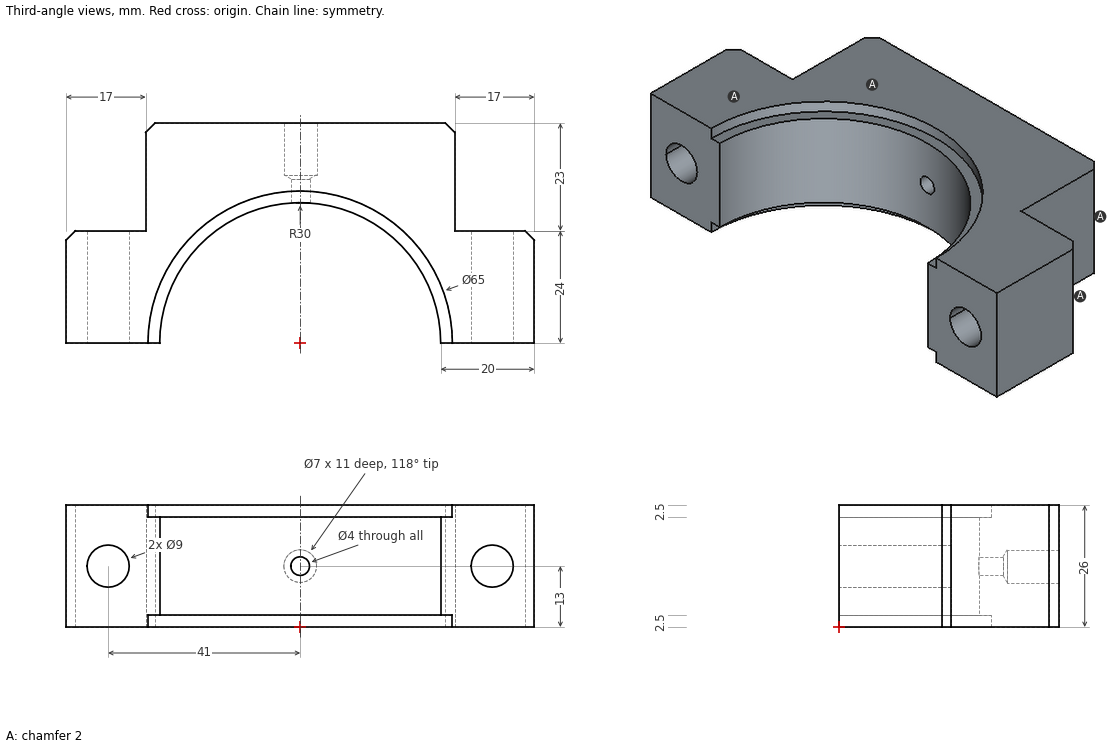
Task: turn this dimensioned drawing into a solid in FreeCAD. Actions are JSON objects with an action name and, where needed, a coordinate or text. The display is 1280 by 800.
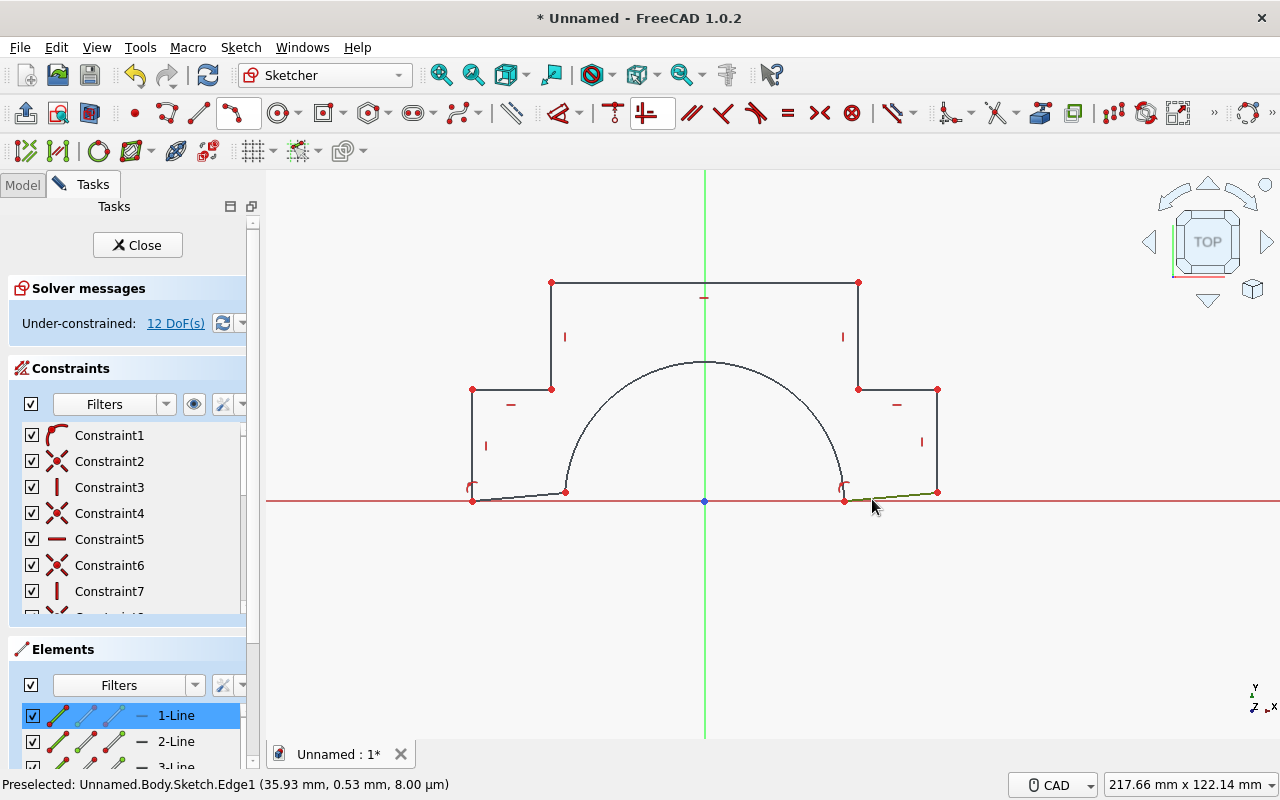
{"action": "key", "text": "h"}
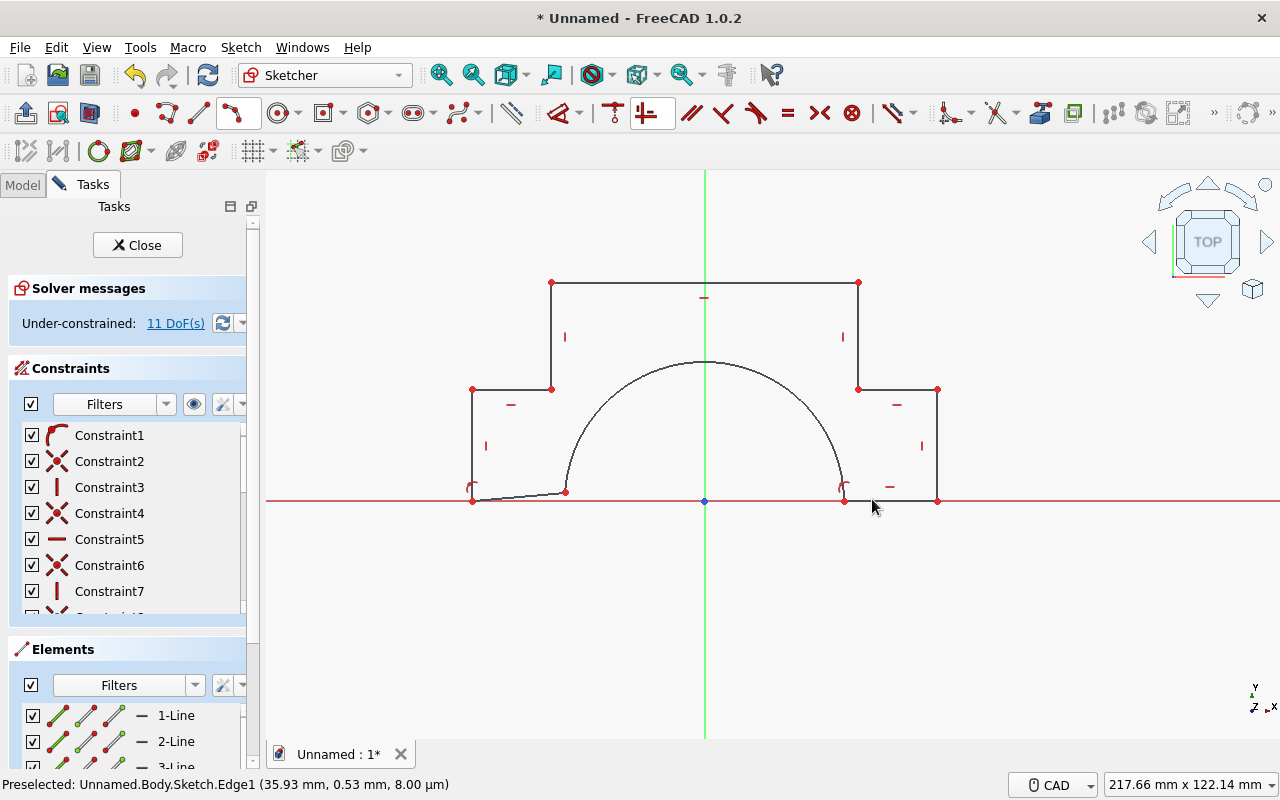
{"action": "left_click", "coordinate": [500, 499]}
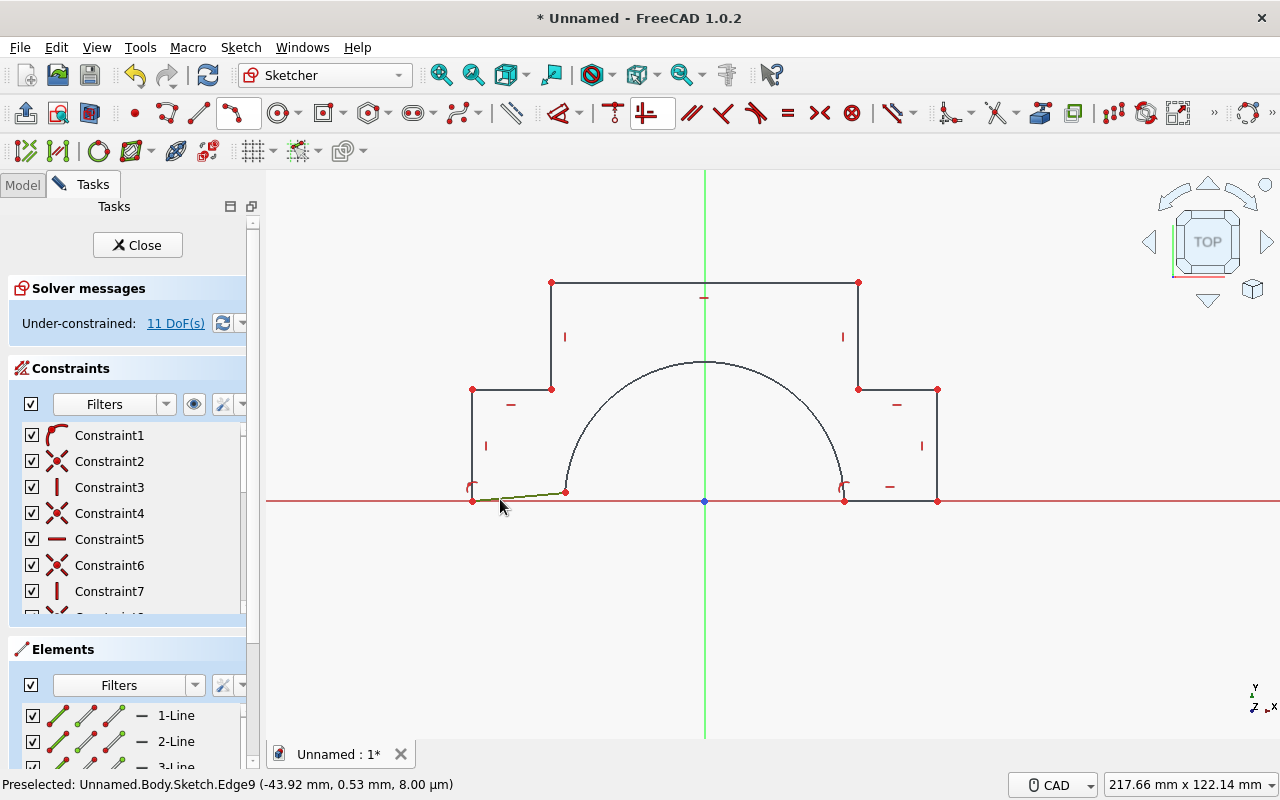
{"action": "key", "text": "h"}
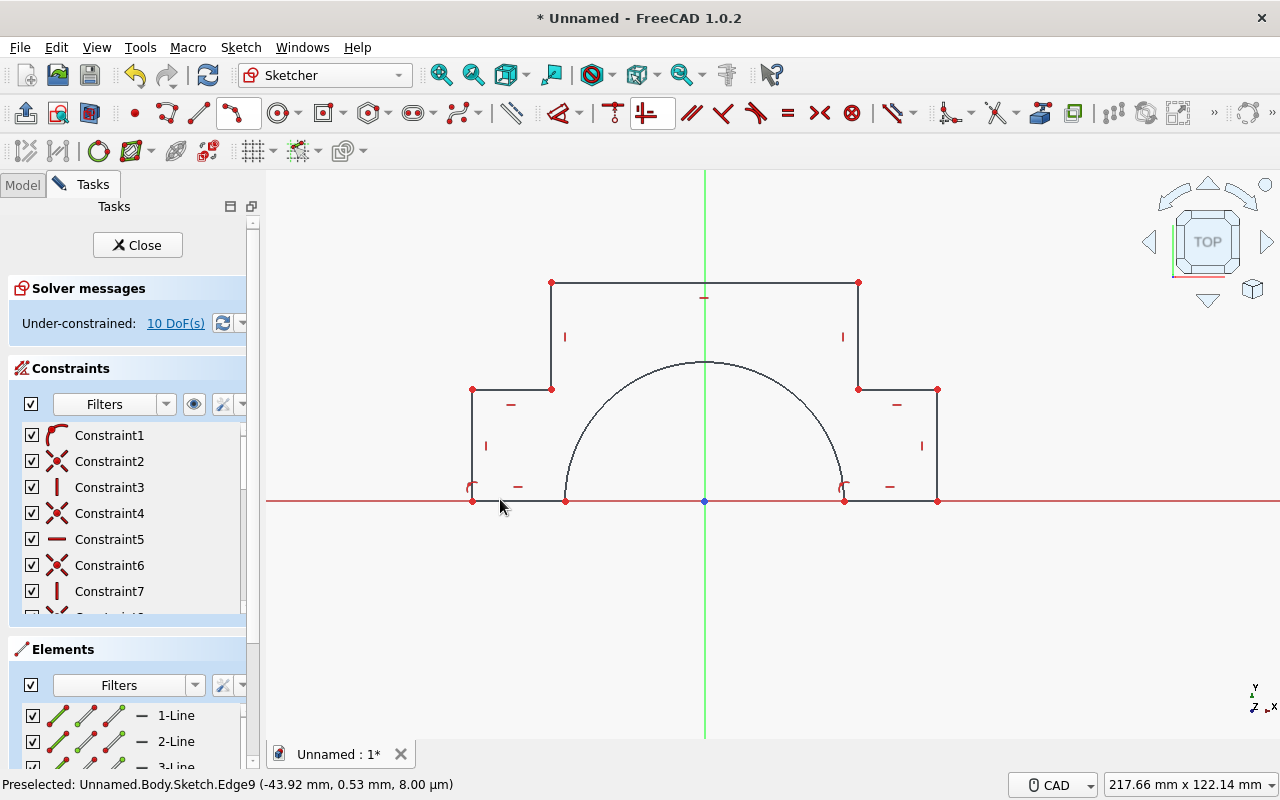
{"action": "left_click_drag", "start_coordinate": [695, 491], "coordinate": [715, 512]}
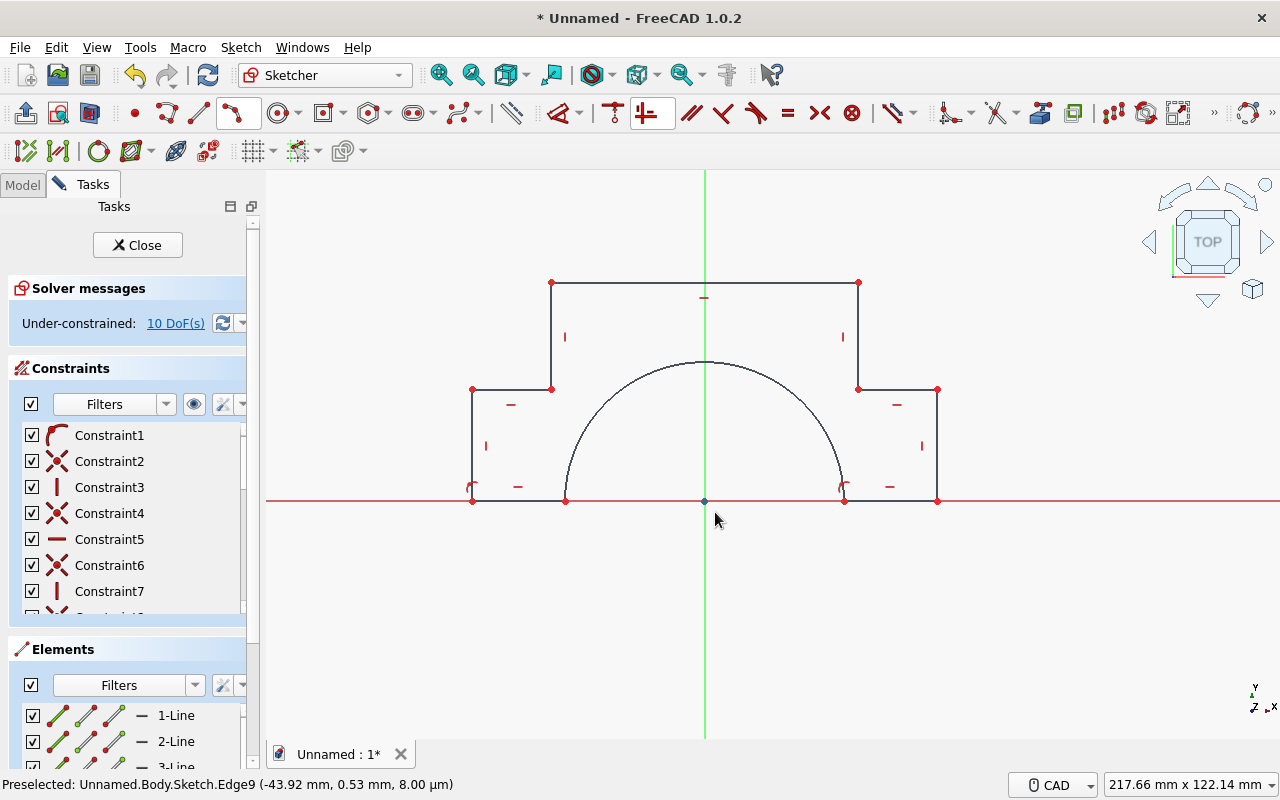
{"action": "key", "text": "c"}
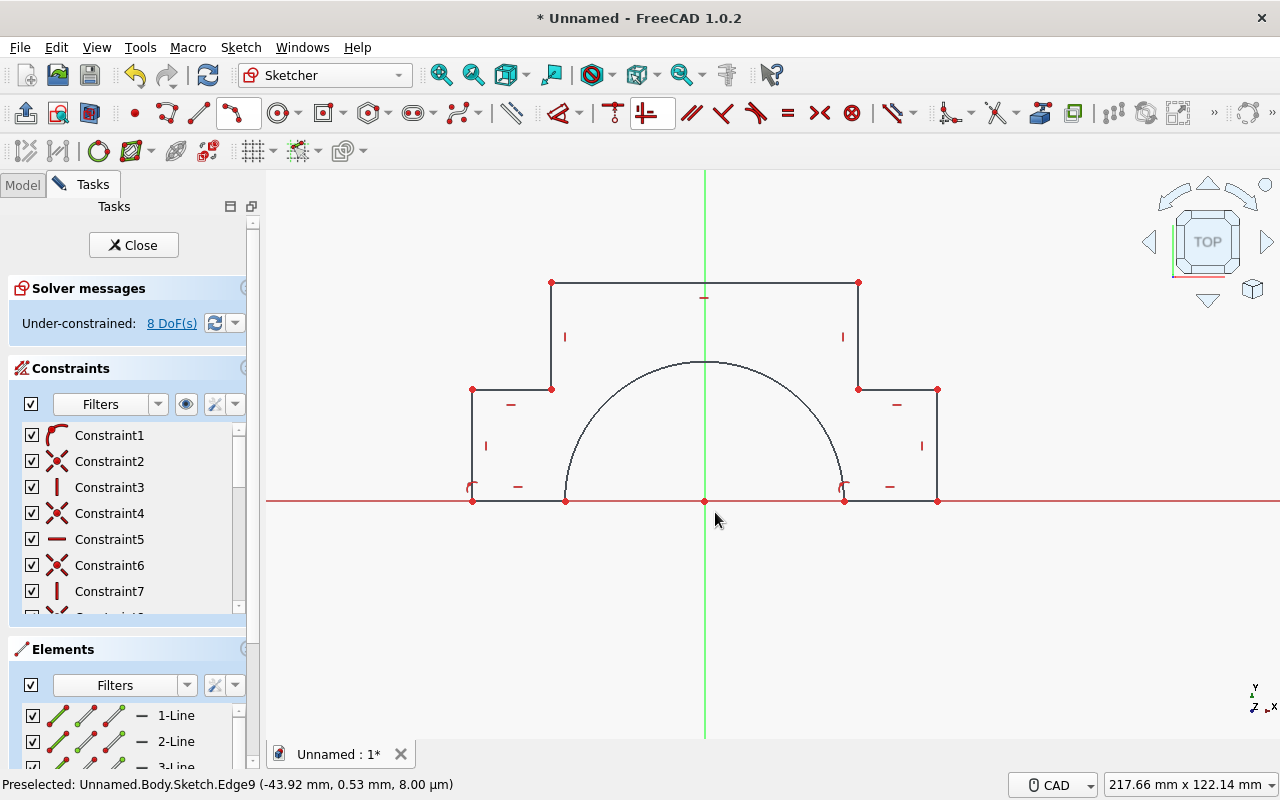
{"action": "left_click", "coordinate": [858, 390]}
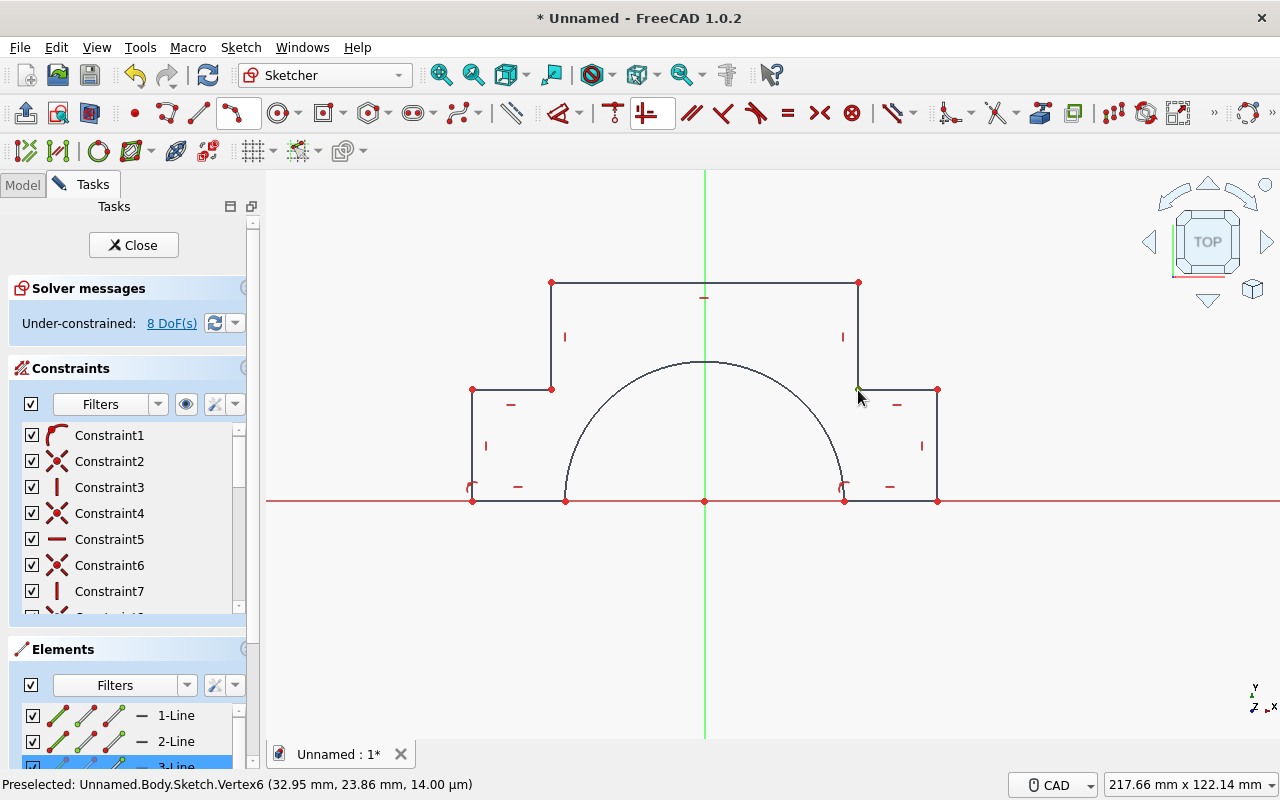
{"action": "left_click", "coordinate": [551, 390]}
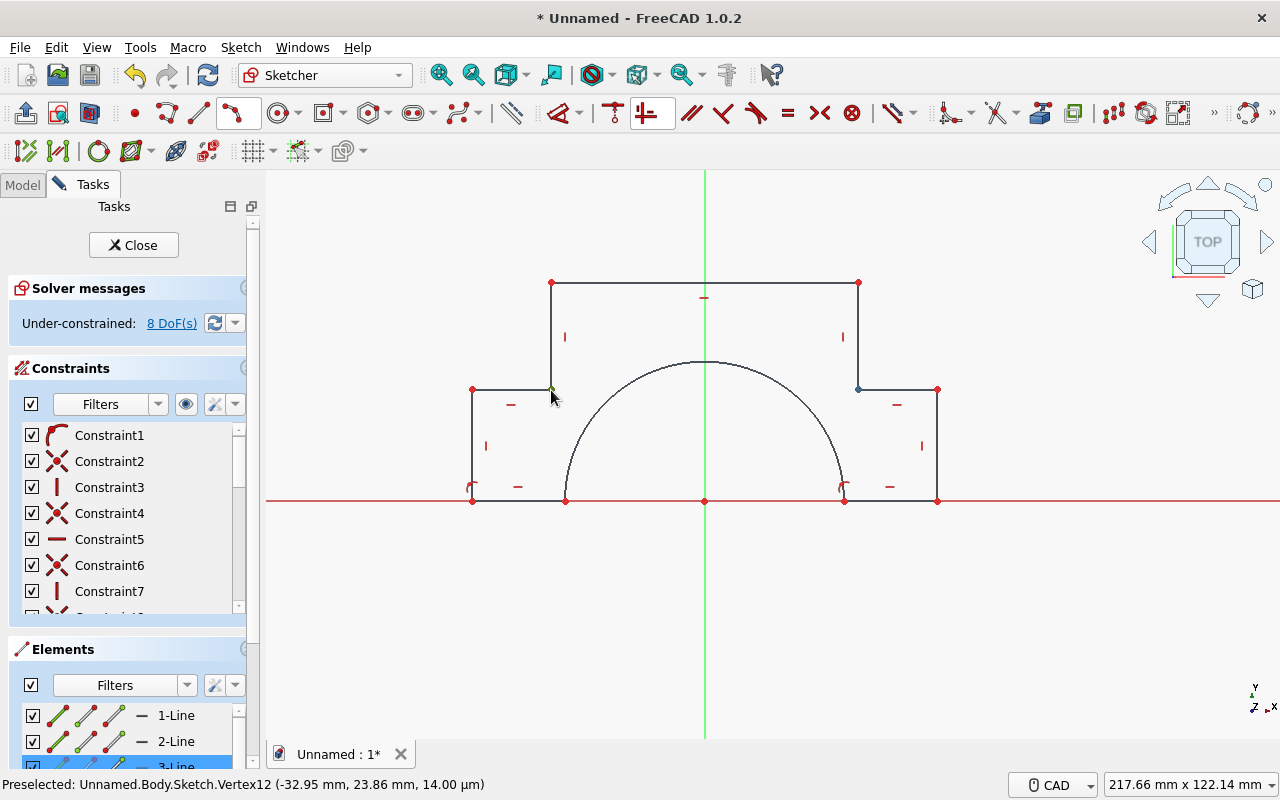
{"action": "left_click", "coordinate": [705, 674]}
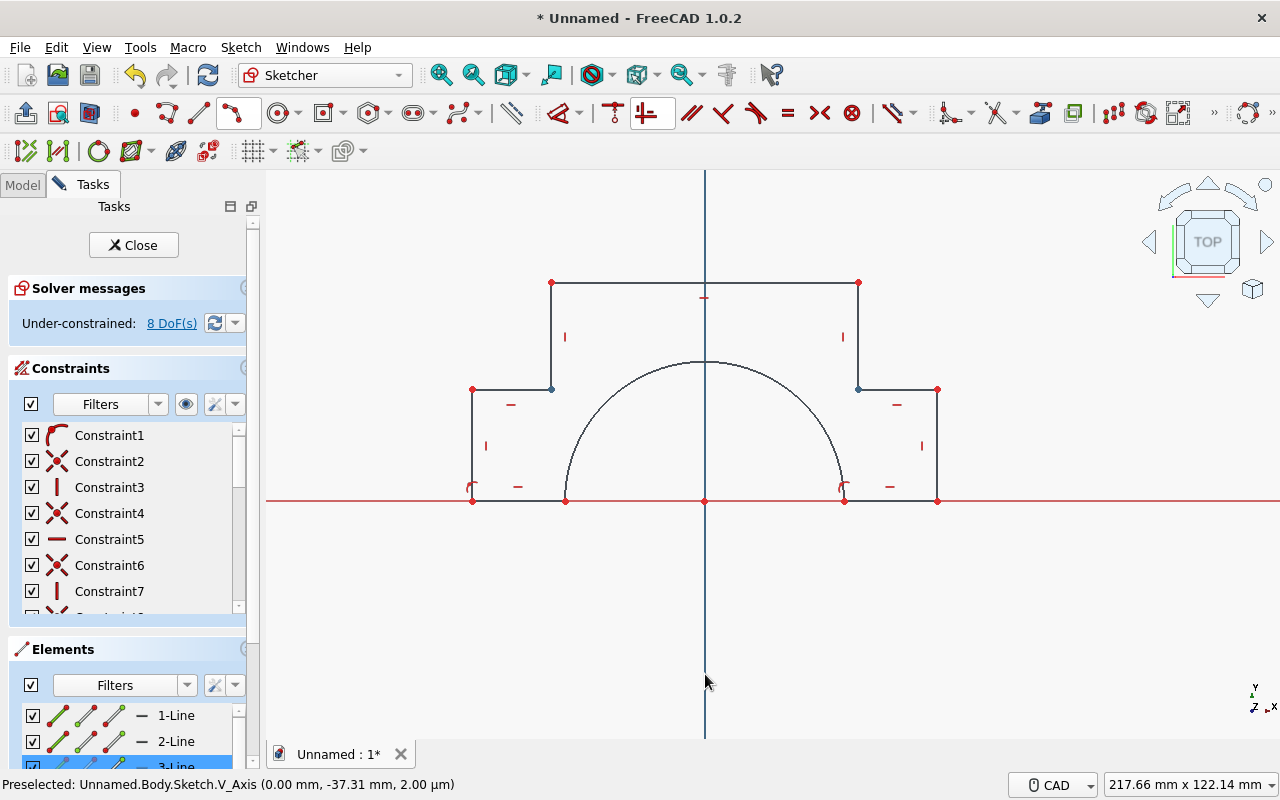
{"action": "key", "text": "s"}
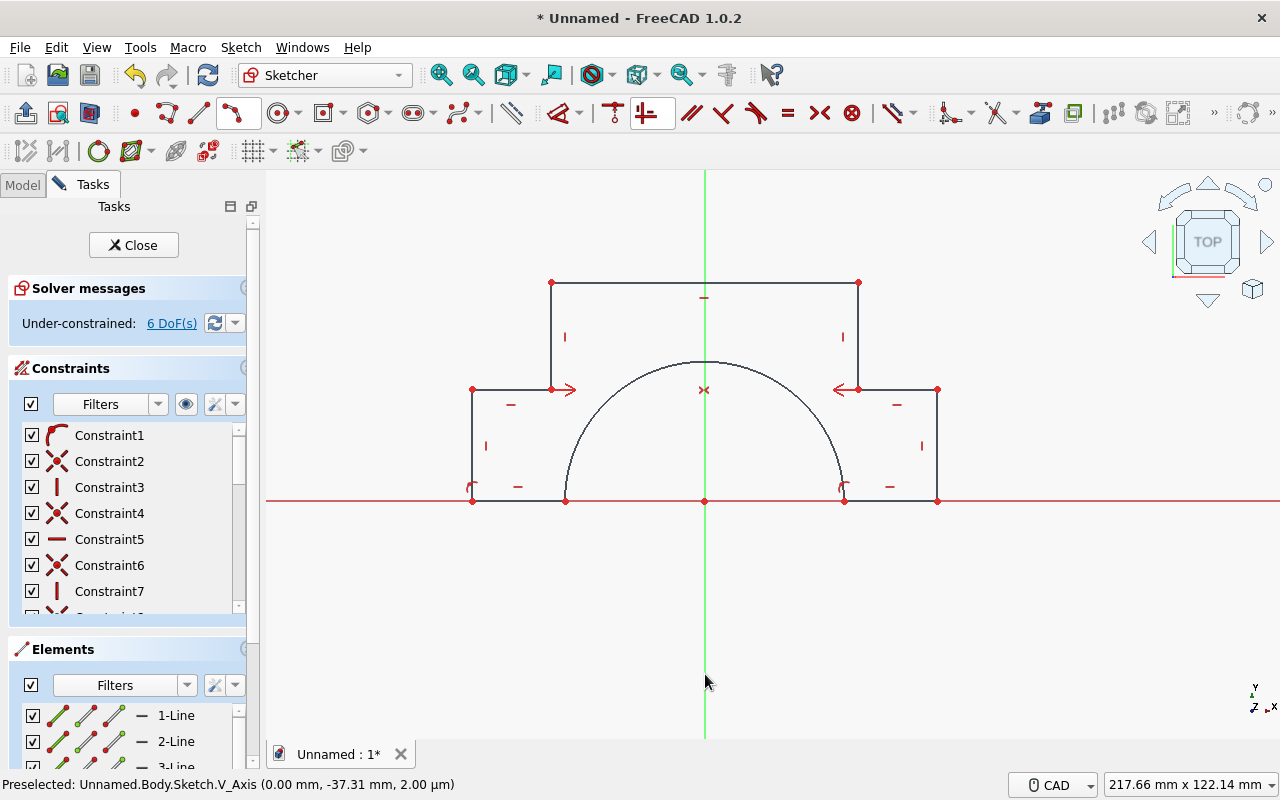
{"action": "left_click", "coordinate": [787, 388]}